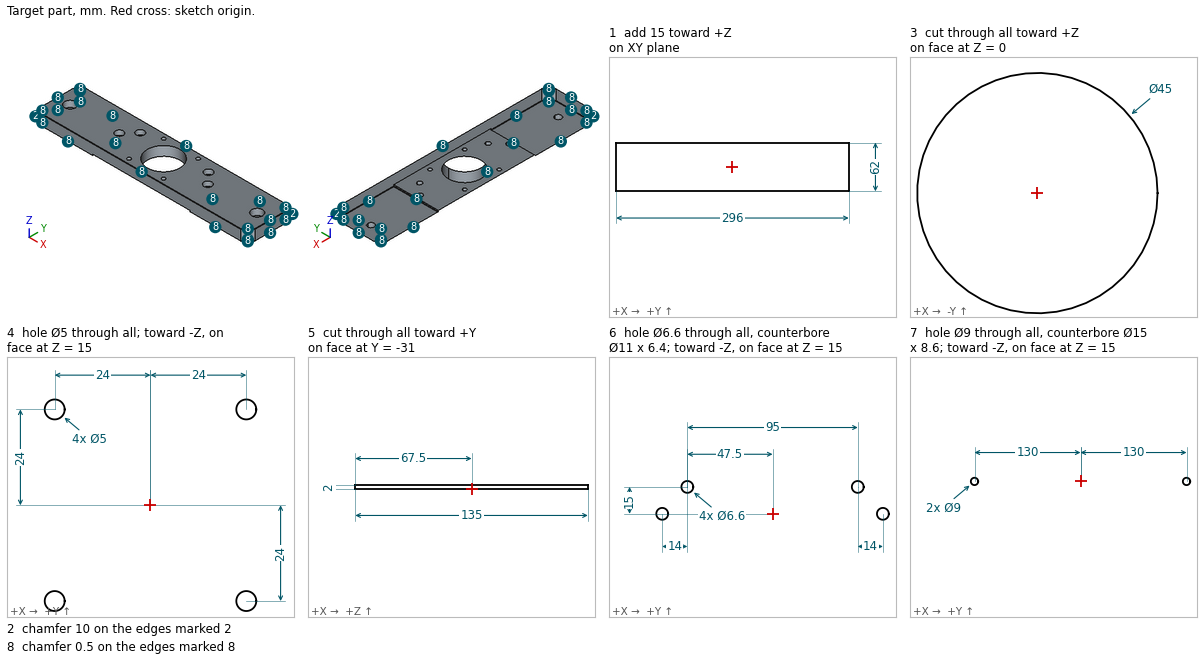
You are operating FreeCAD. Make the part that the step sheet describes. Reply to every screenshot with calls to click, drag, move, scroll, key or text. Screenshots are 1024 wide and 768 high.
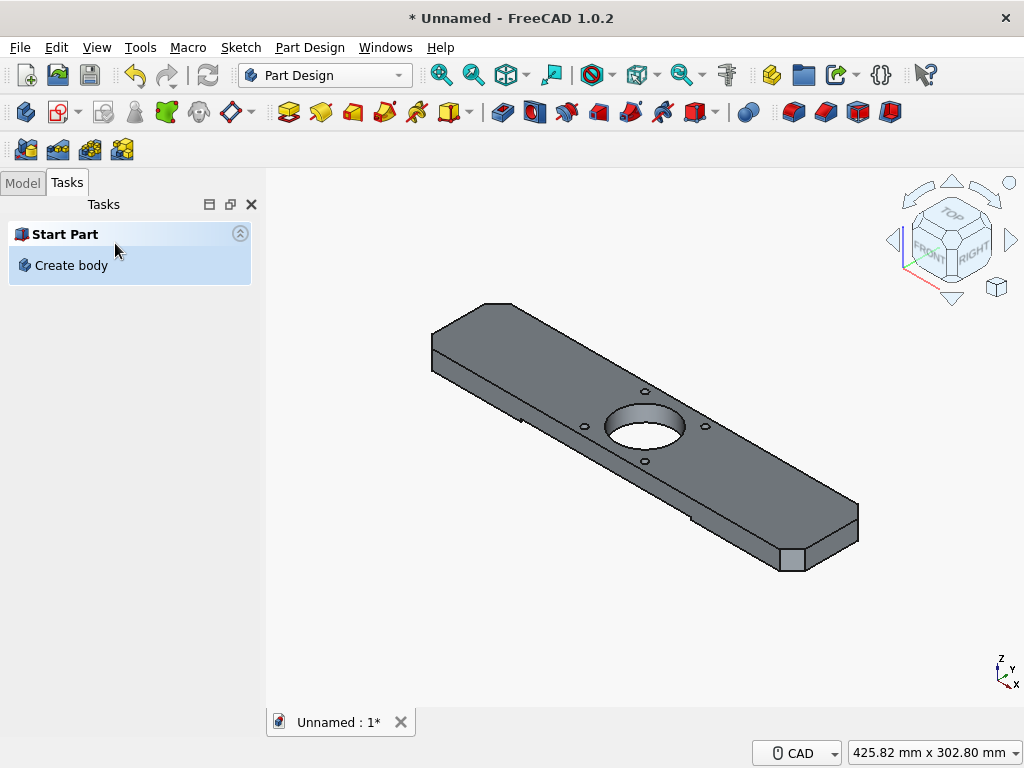
click(751, 487)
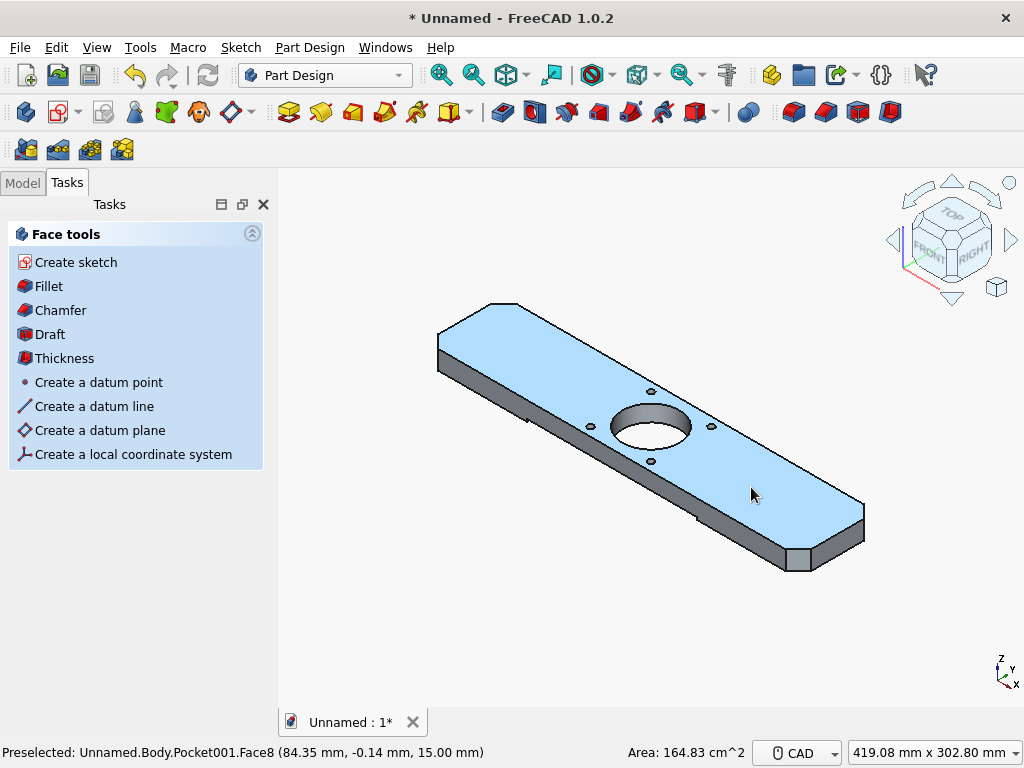
click(58, 112)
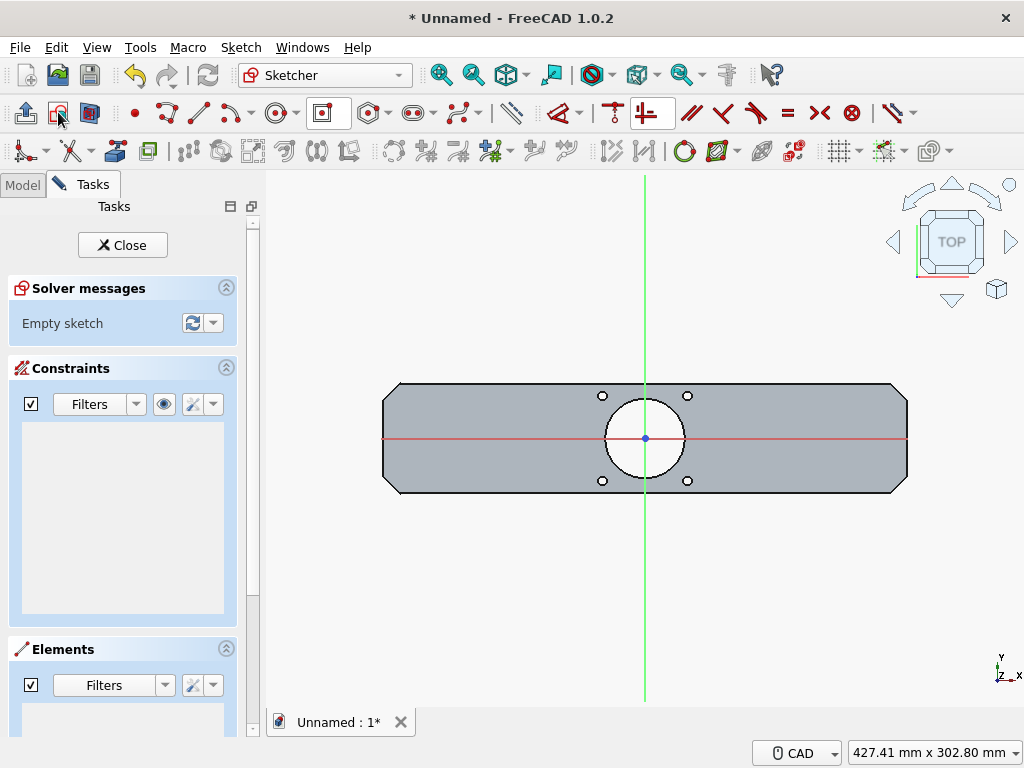
scroll(728, 409, up, 3)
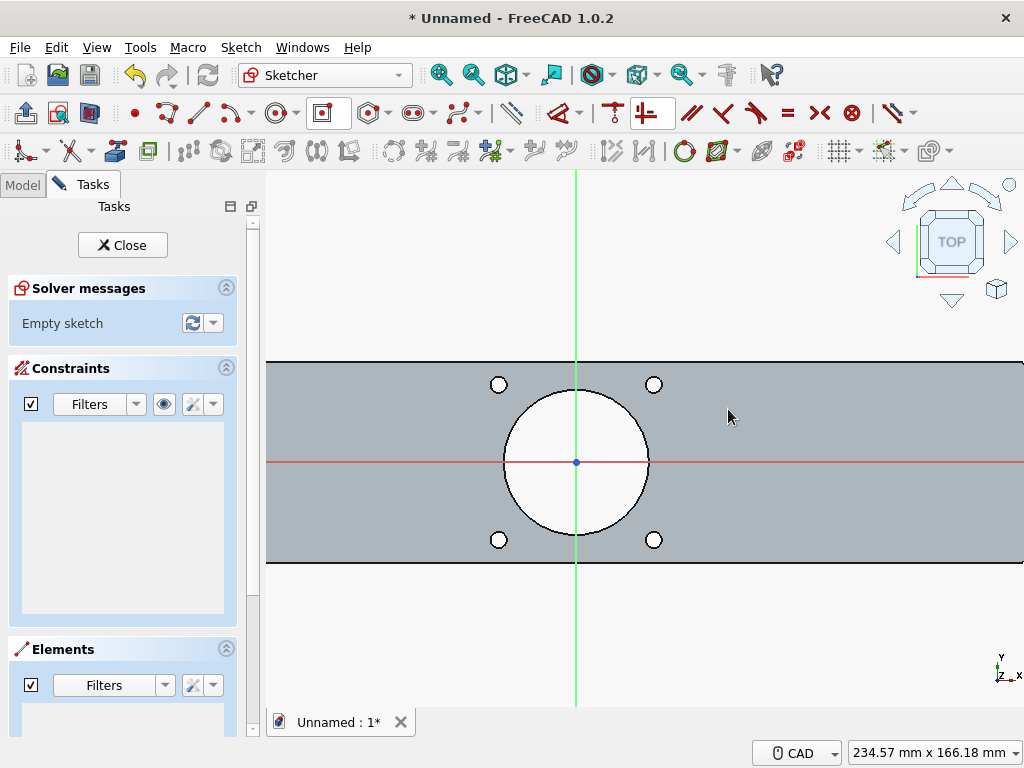
click(276, 114)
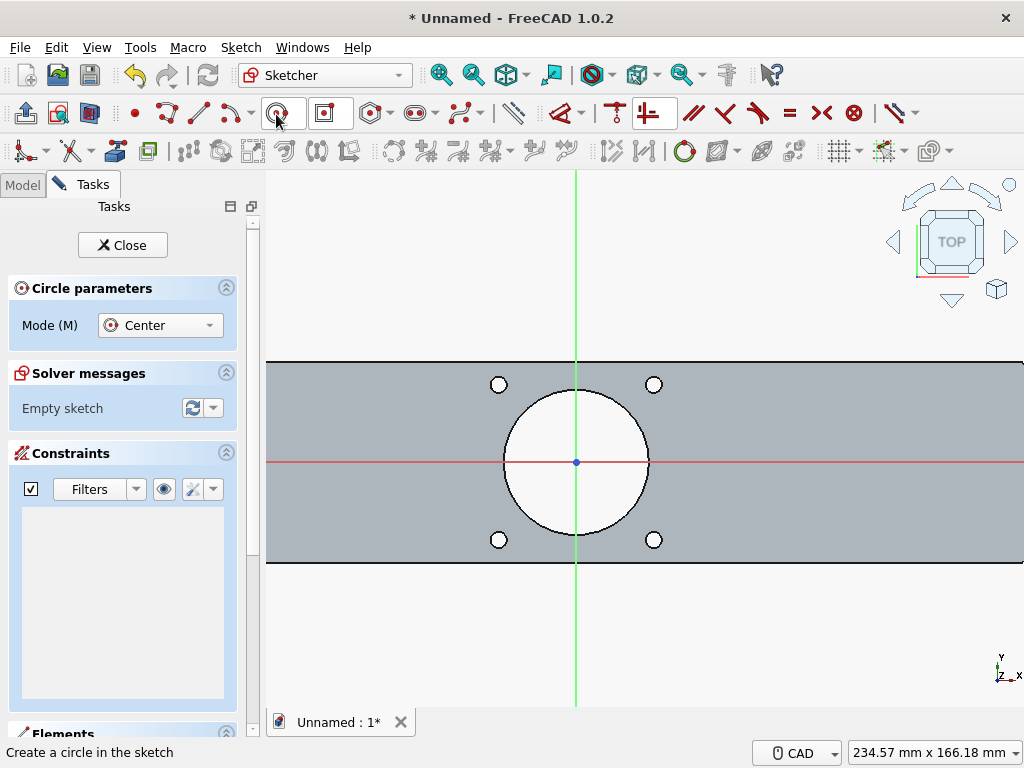
scroll(423, 414, up, 4)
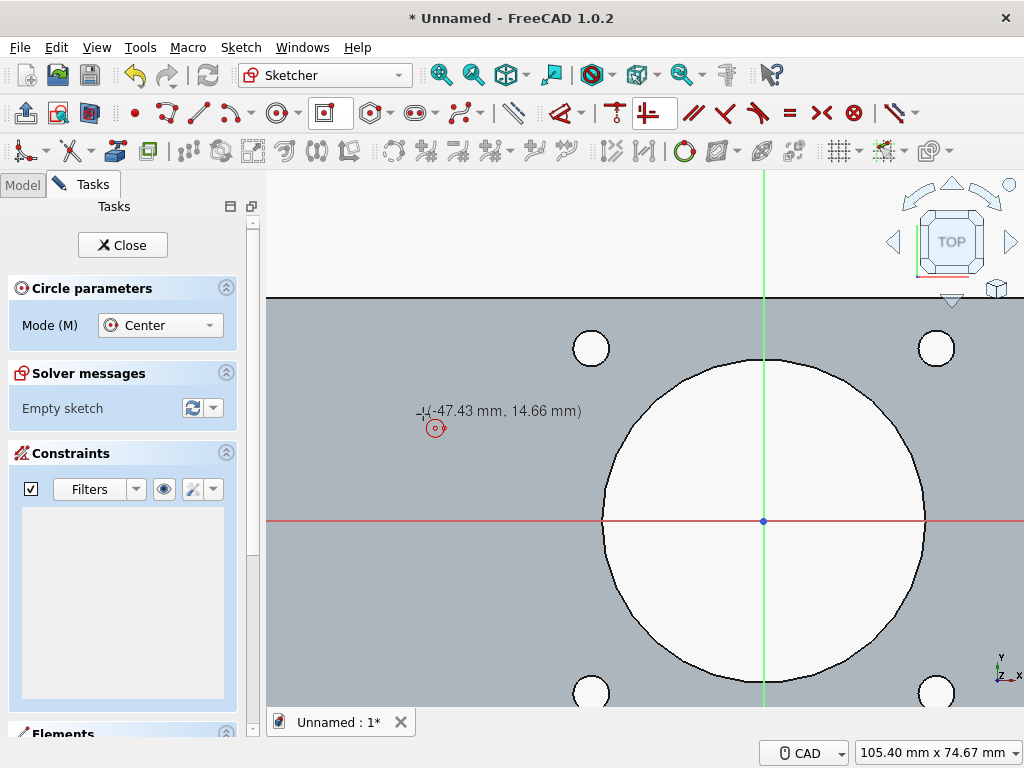
click(422, 413)
move(439, 396)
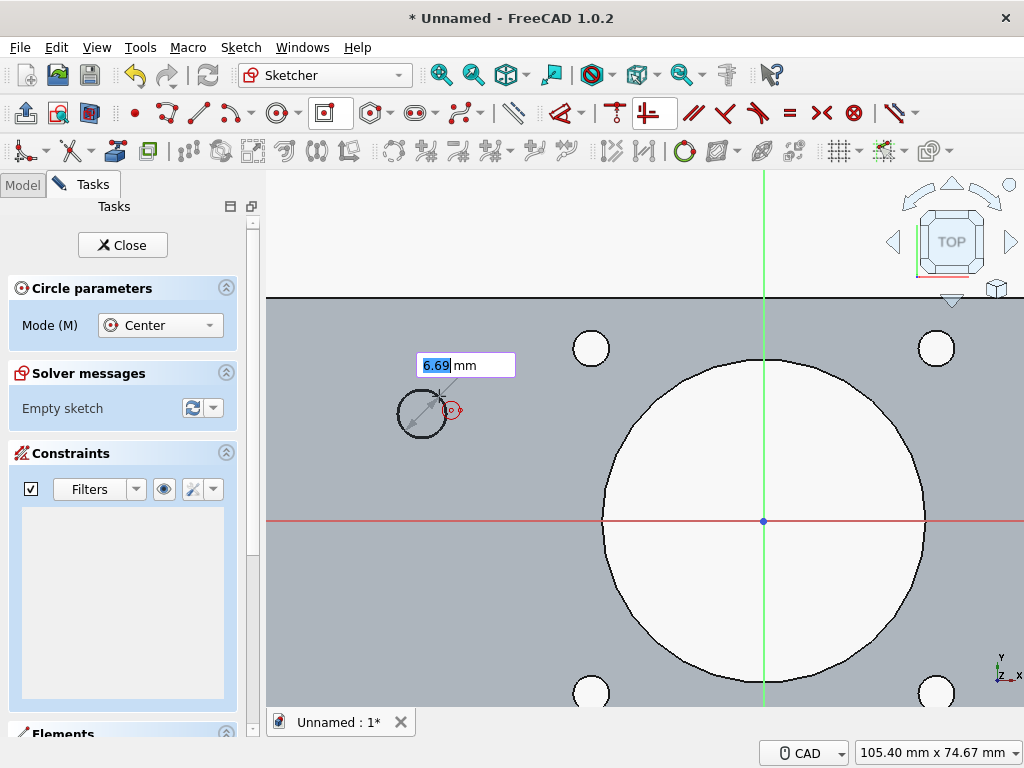
text(6.6)
key(Return)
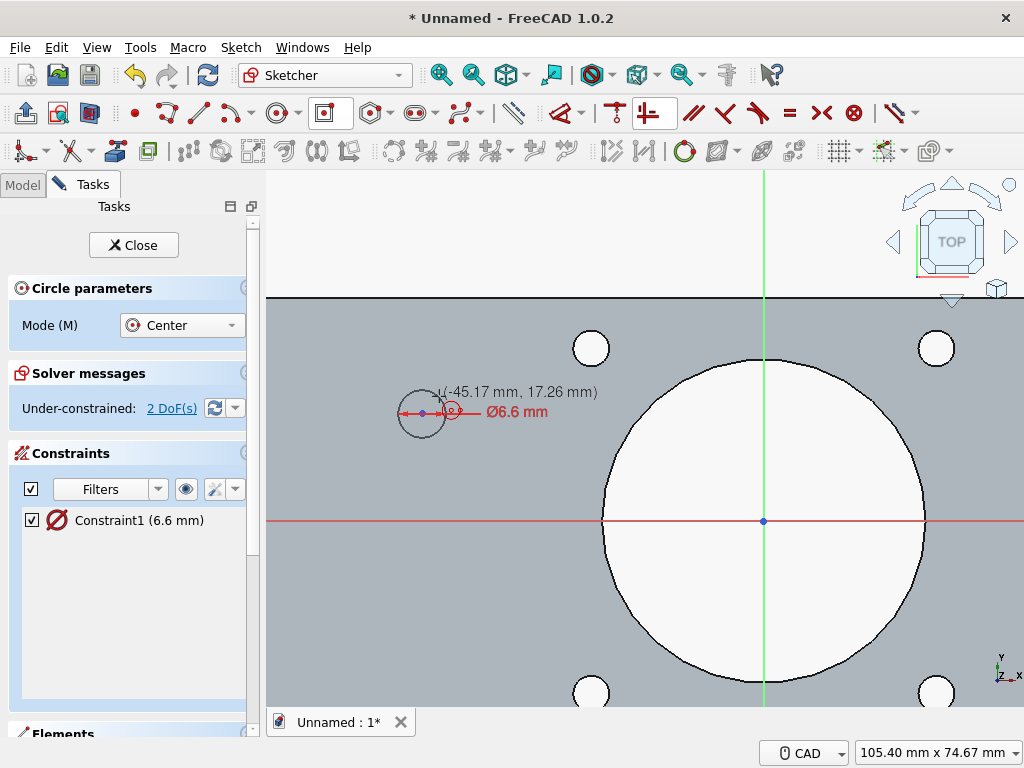
click(322, 521)
move(338, 504)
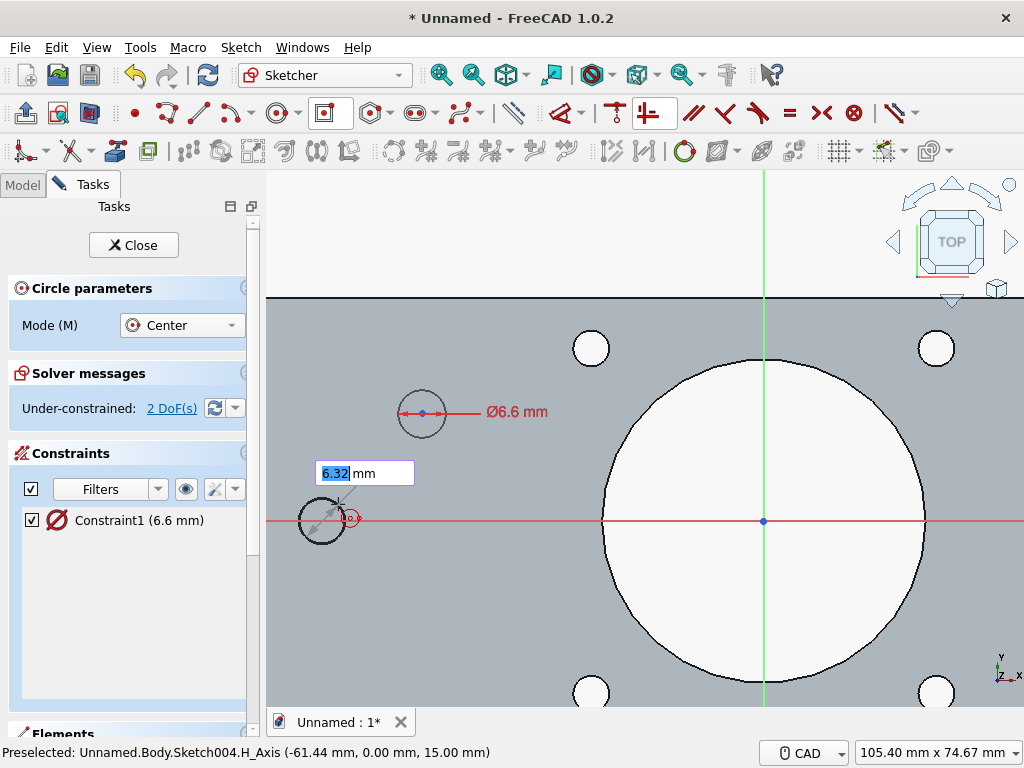
text(6.6)
key(Return)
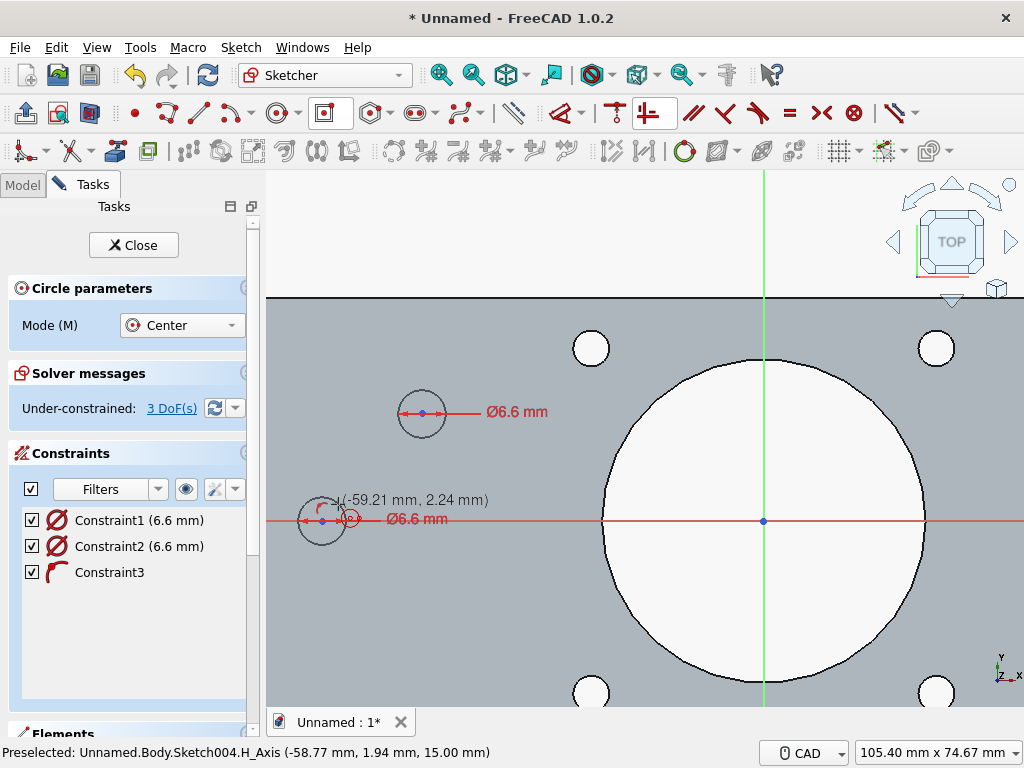
scroll(424, 415, down, 4)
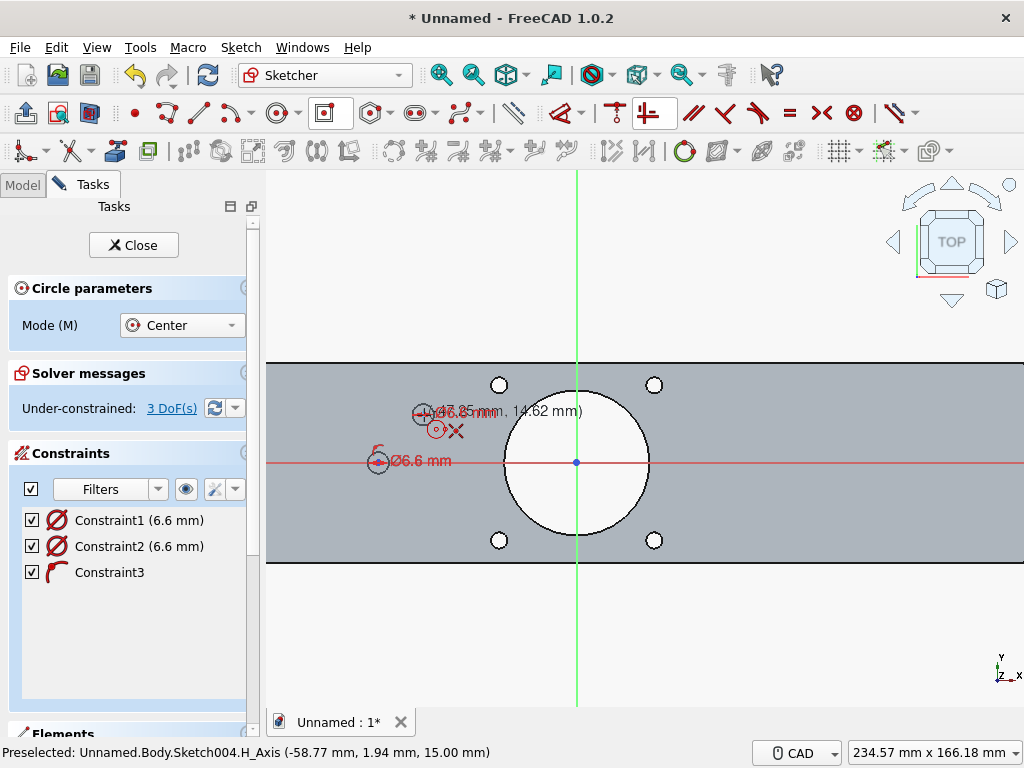
scroll(730, 414, up, 4)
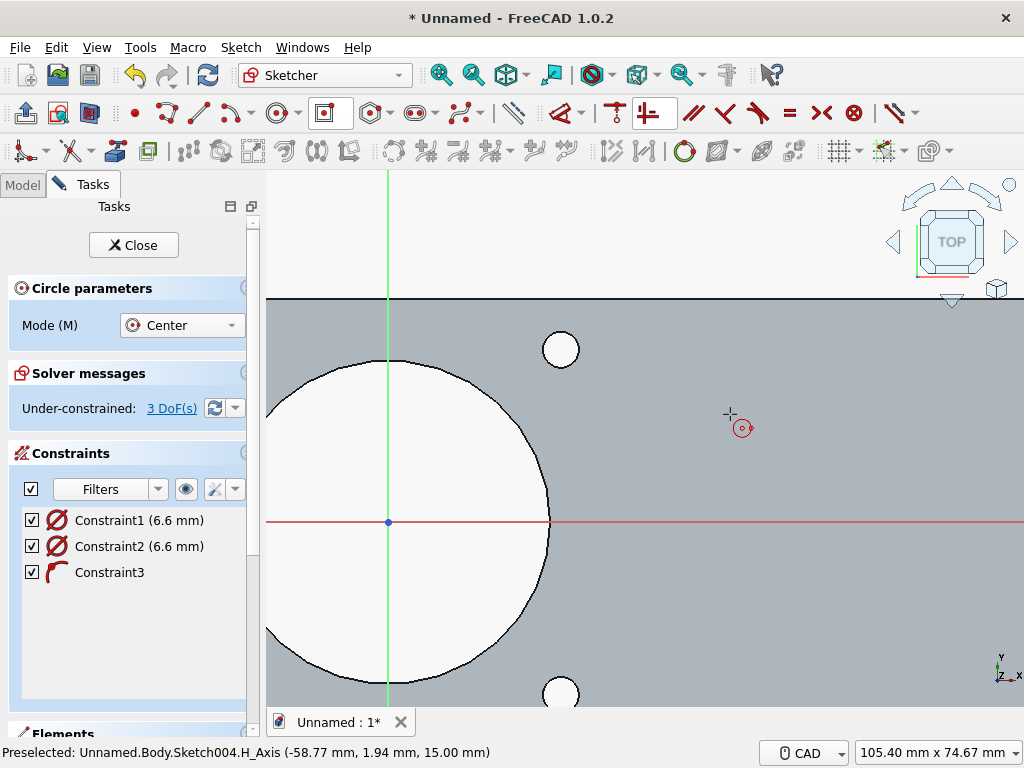
click(730, 414)
move(747, 398)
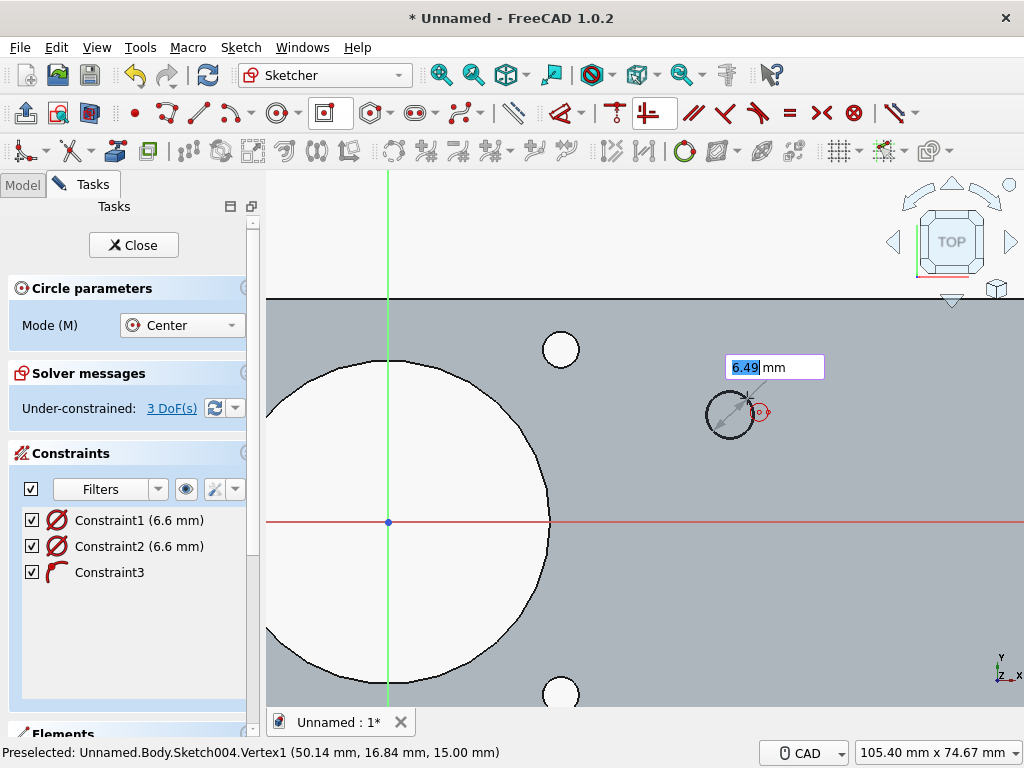
text(6.6)
key(Return)